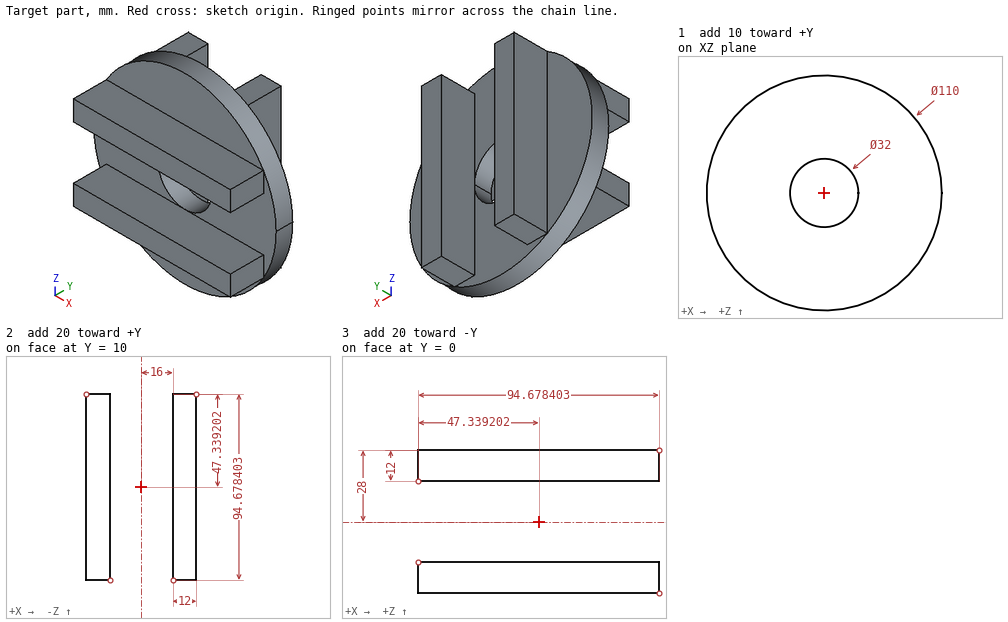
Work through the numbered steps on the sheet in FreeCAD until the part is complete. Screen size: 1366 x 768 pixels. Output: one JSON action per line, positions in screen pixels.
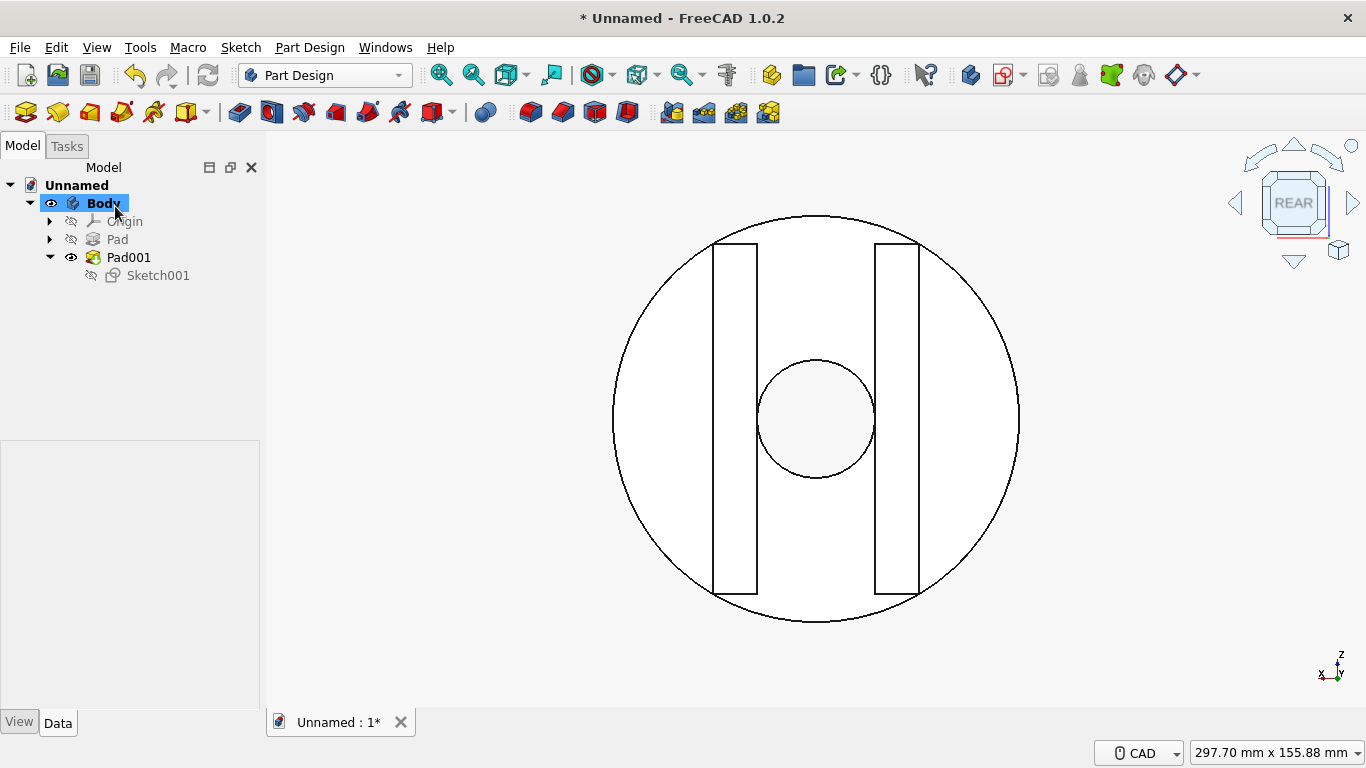
{"action": "key", "text": "0"}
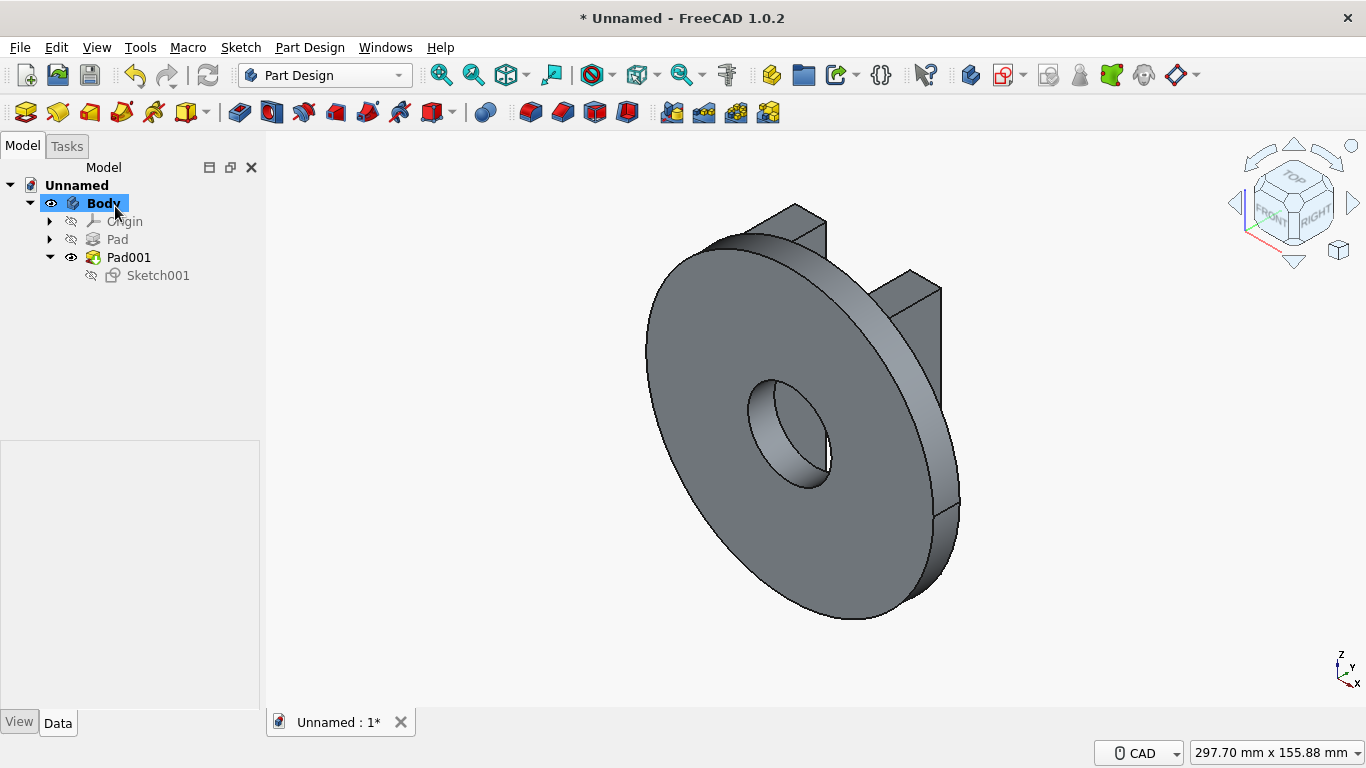
{"action": "left_click", "coordinate": [749, 315]}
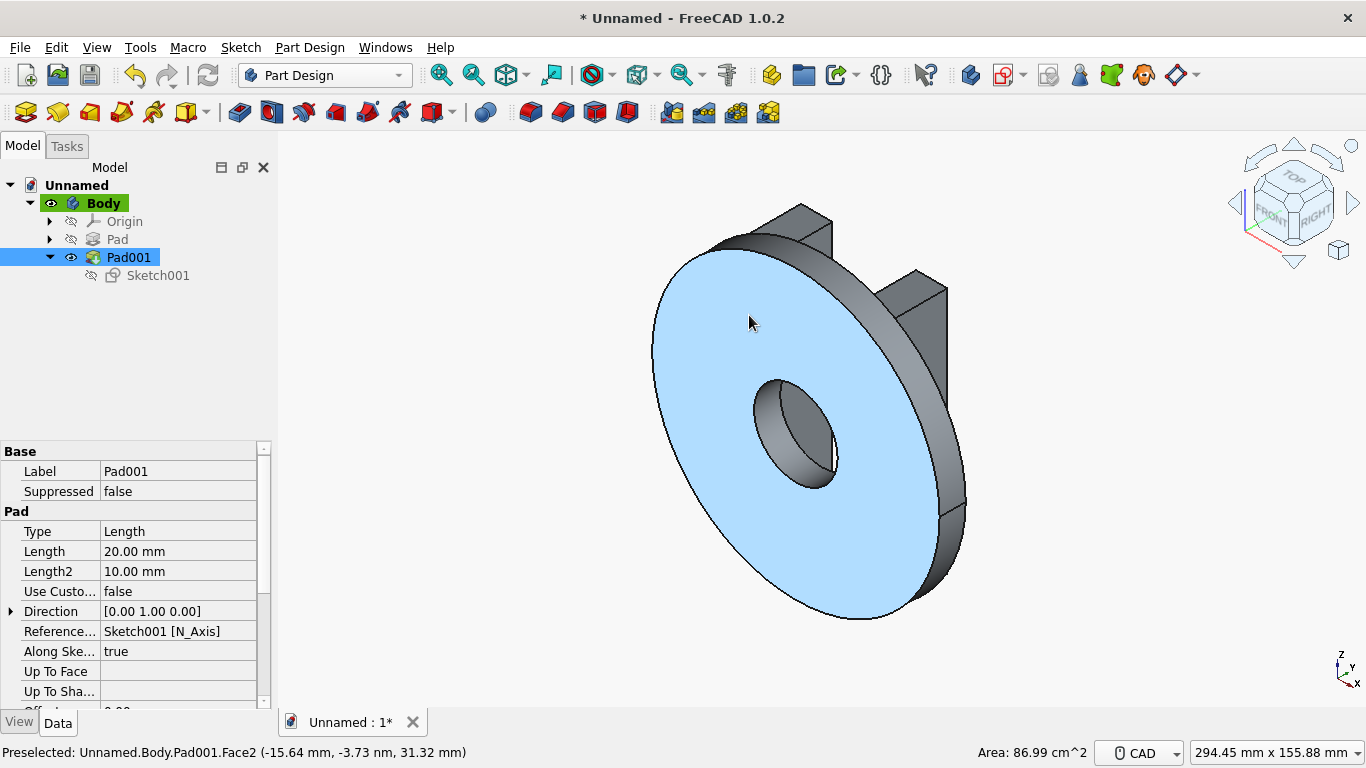
{"action": "left_click", "coordinate": [1004, 76]}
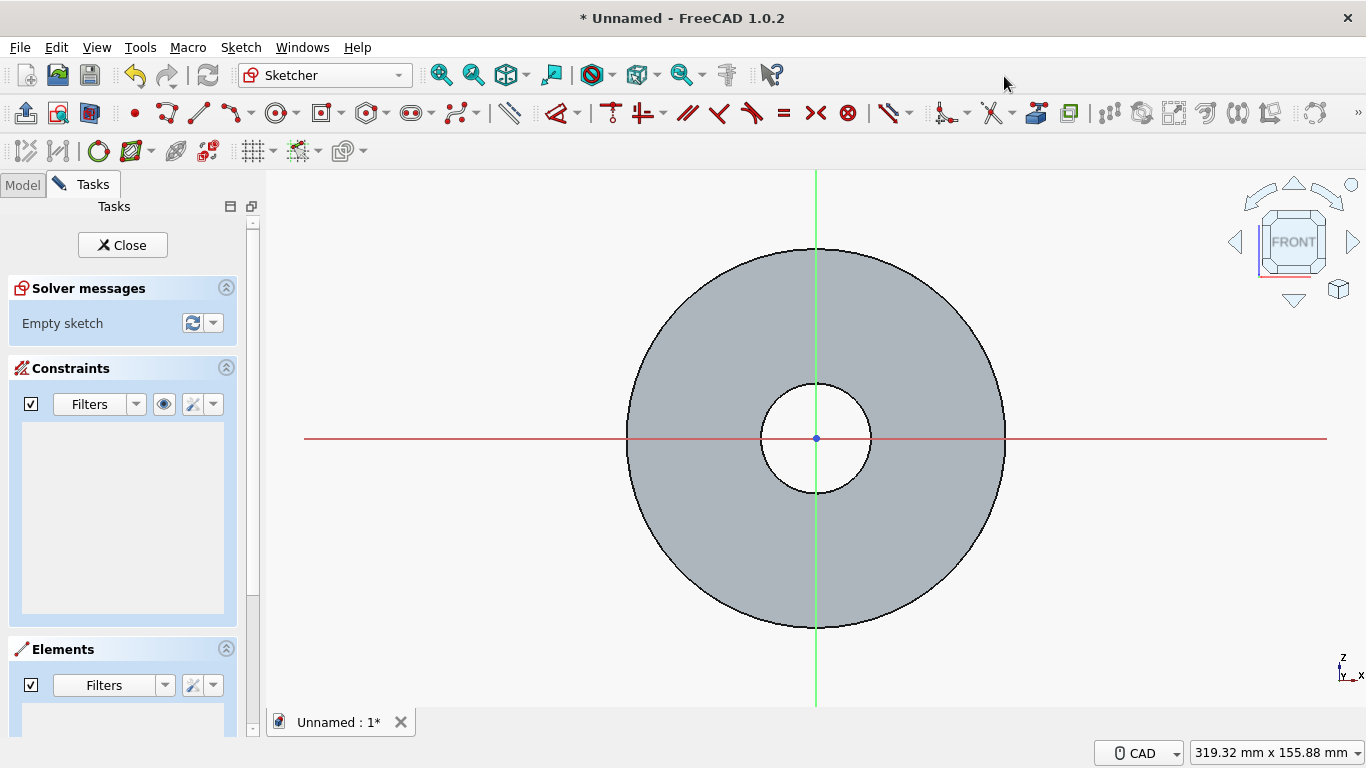
{"action": "scroll", "coordinate": [899, 439], "scroll_direction": "up", "scroll_amount": 3}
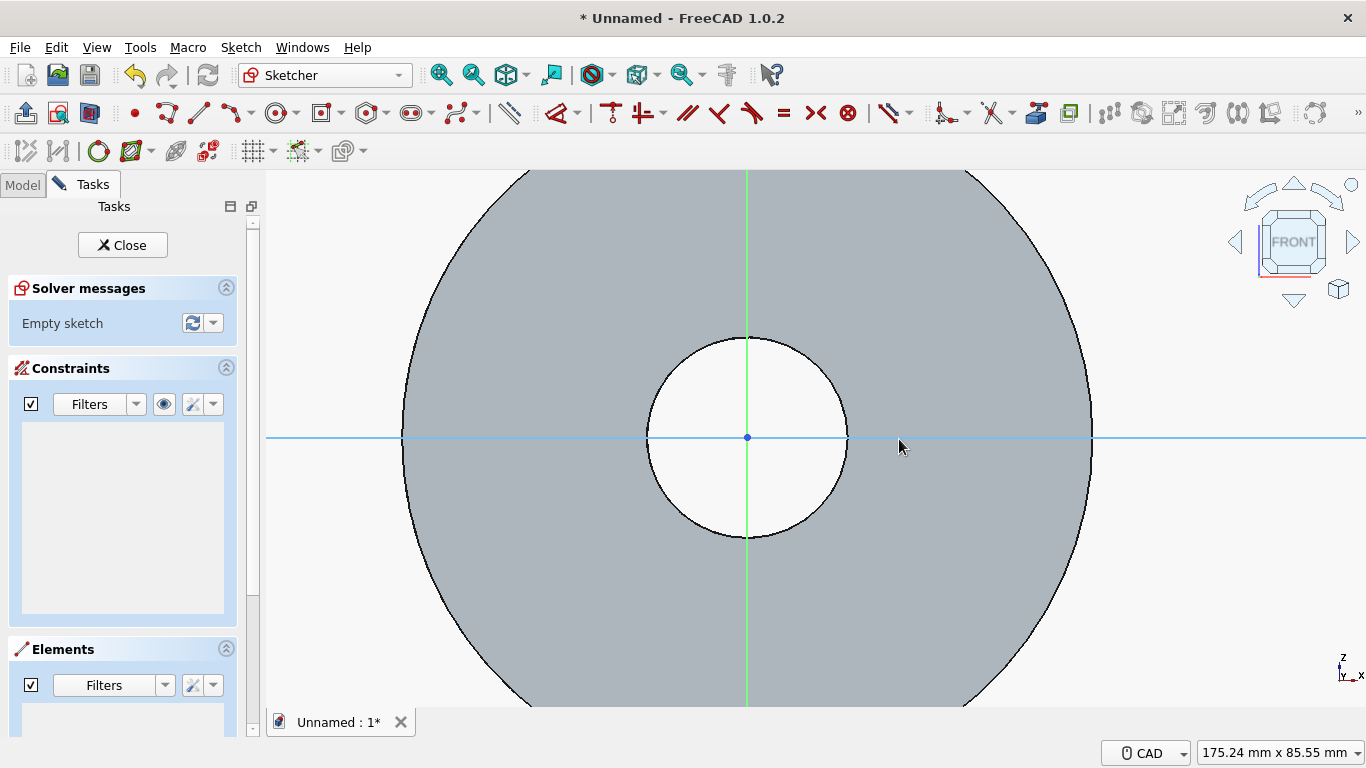
{"action": "key", "text": "g r"}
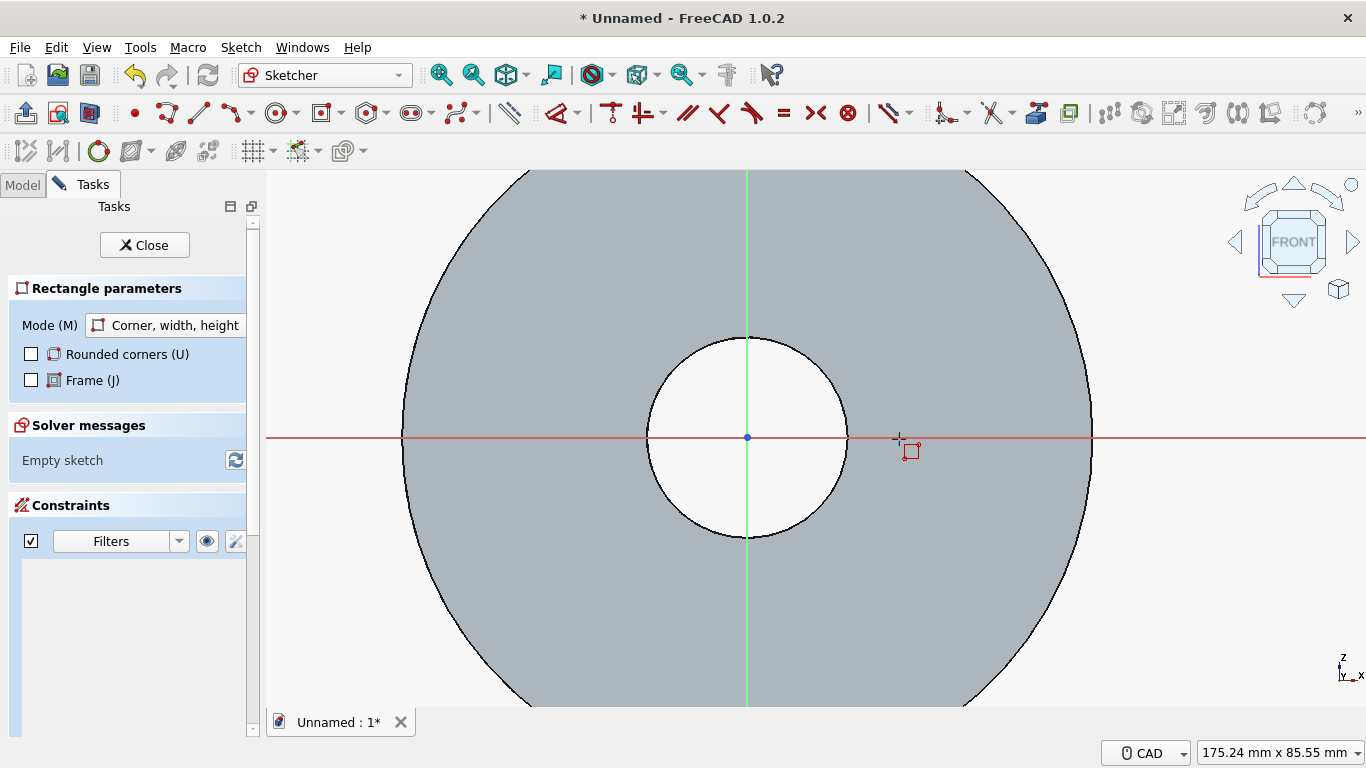
{"action": "left_click", "coordinate": [450, 262]}
{"action": "left_click", "coordinate": [1044, 337]}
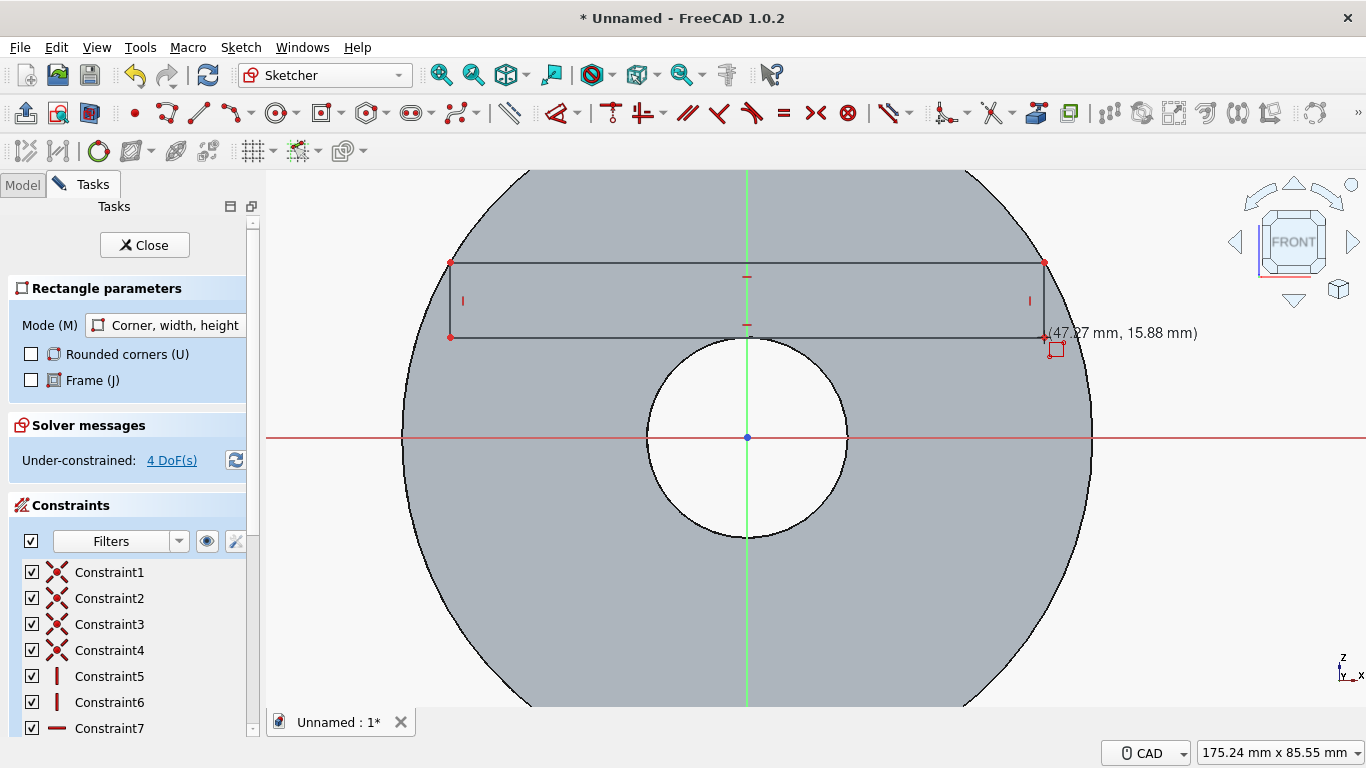
{"action": "left_click", "coordinate": [450, 538]}
{"action": "left_click", "coordinate": [1044, 613]}
{"action": "key", "text": "Escape"}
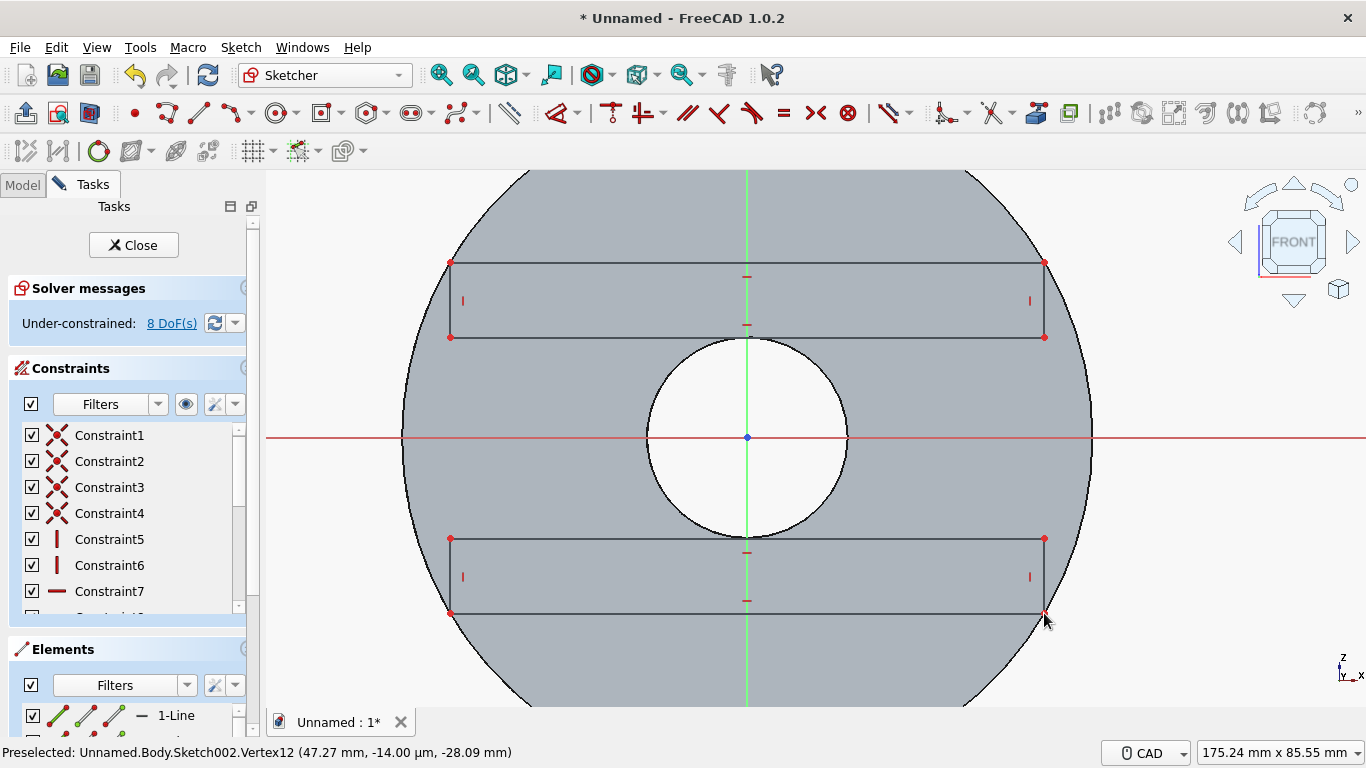
{"action": "left_click", "coordinate": [450, 338]}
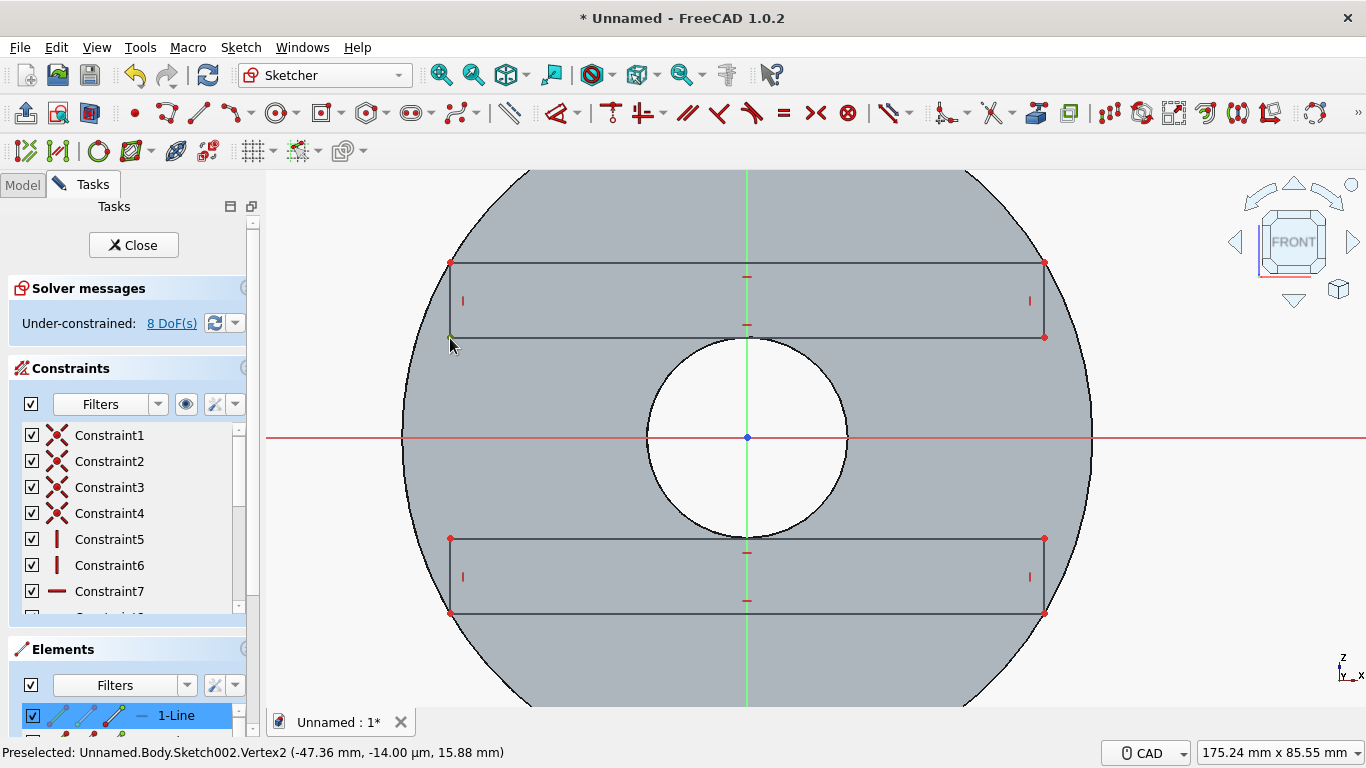
{"action": "left_click", "coordinate": [450, 539]}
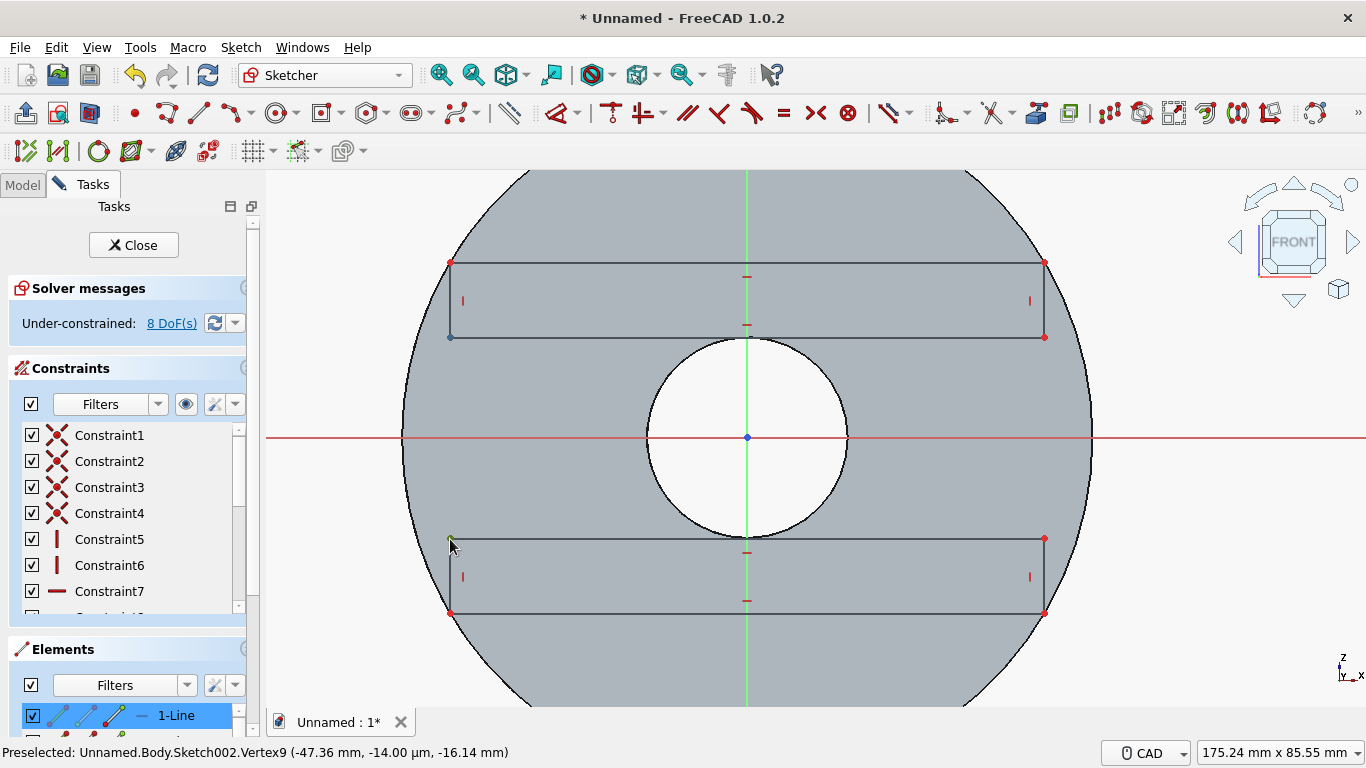
{"action": "left_click", "coordinate": [359, 438]}